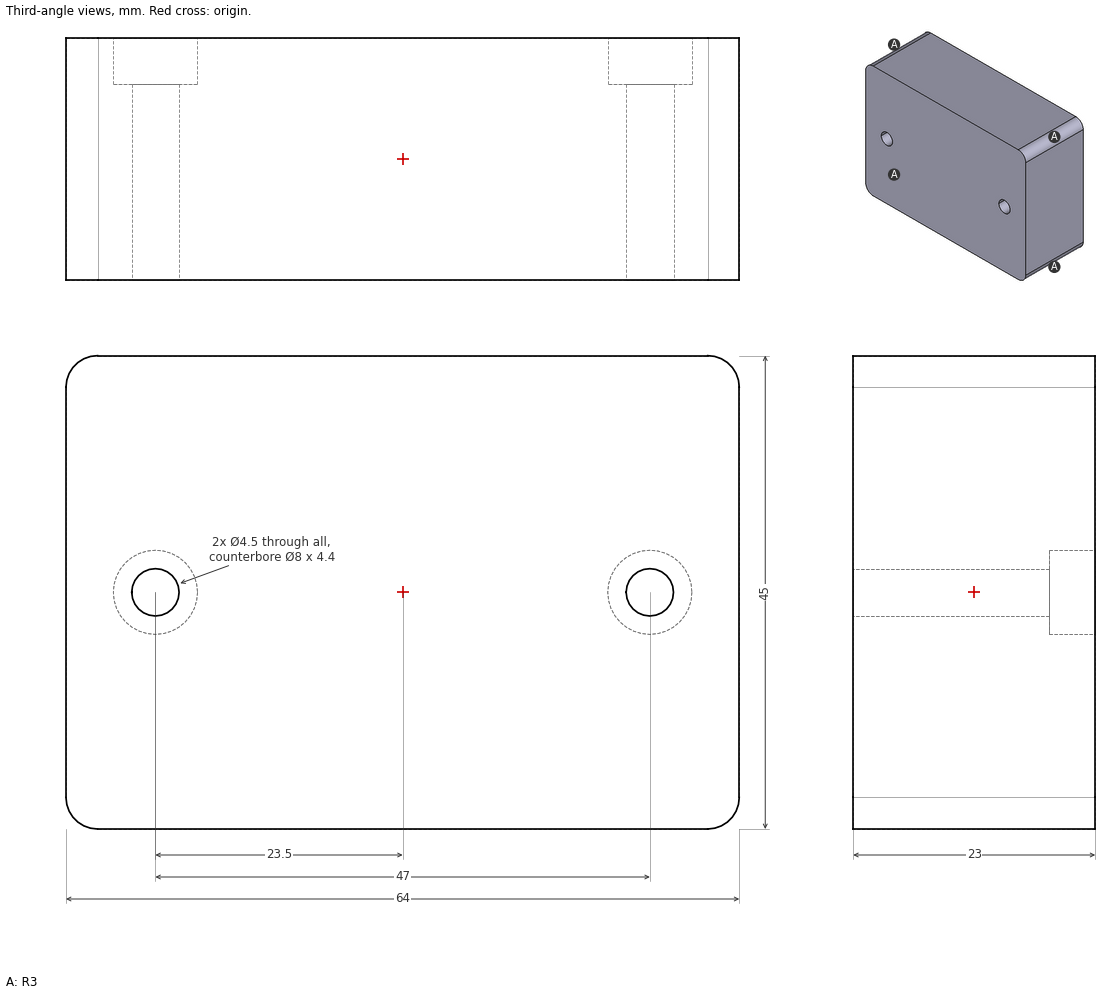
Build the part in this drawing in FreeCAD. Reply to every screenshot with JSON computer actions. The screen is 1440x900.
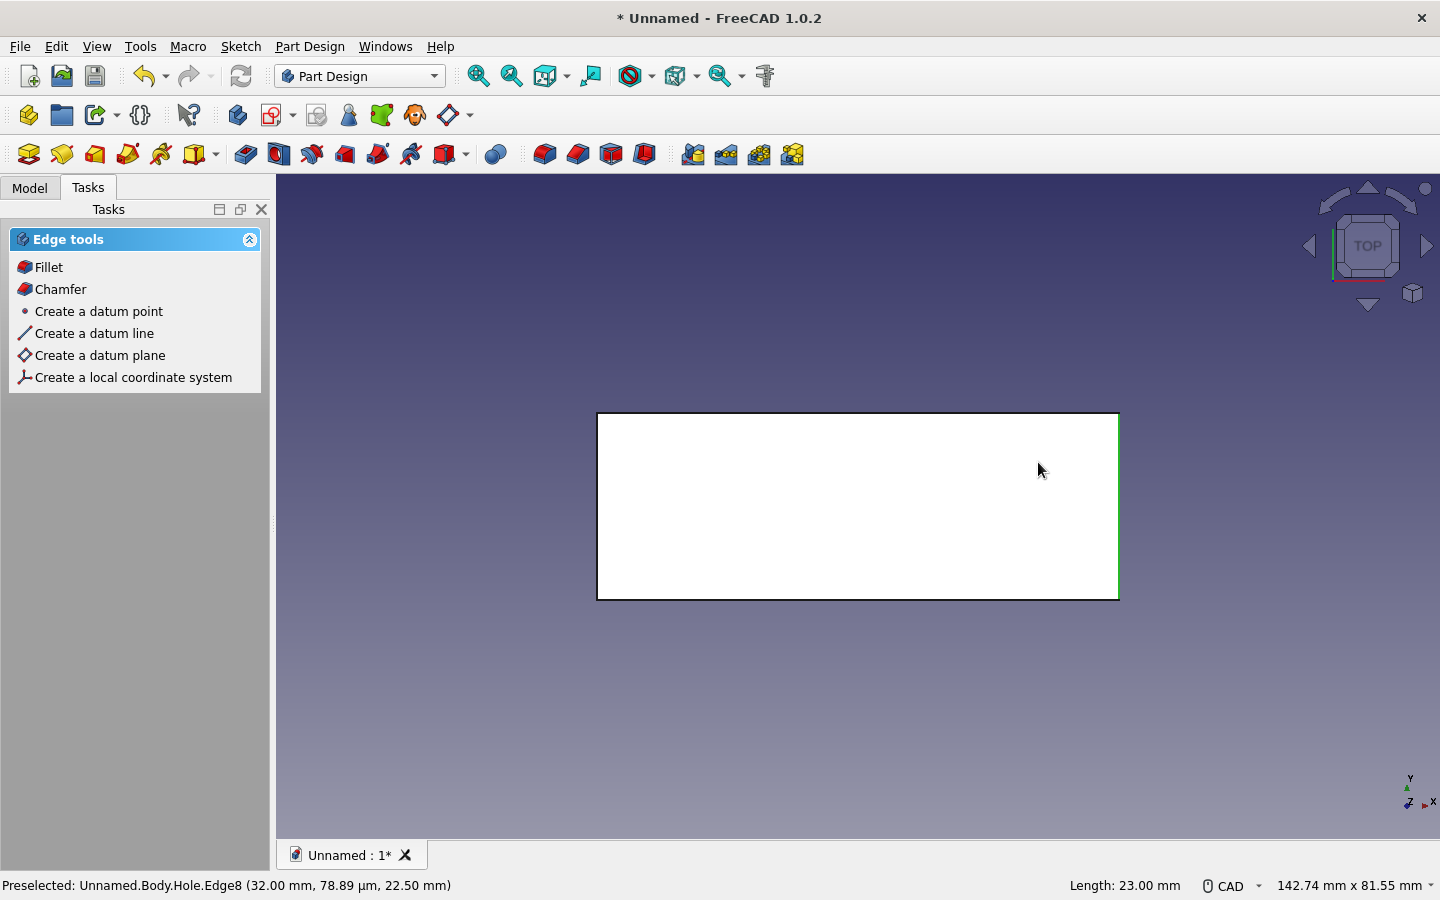
{"action": "left_click", "coordinate": [479, 76]}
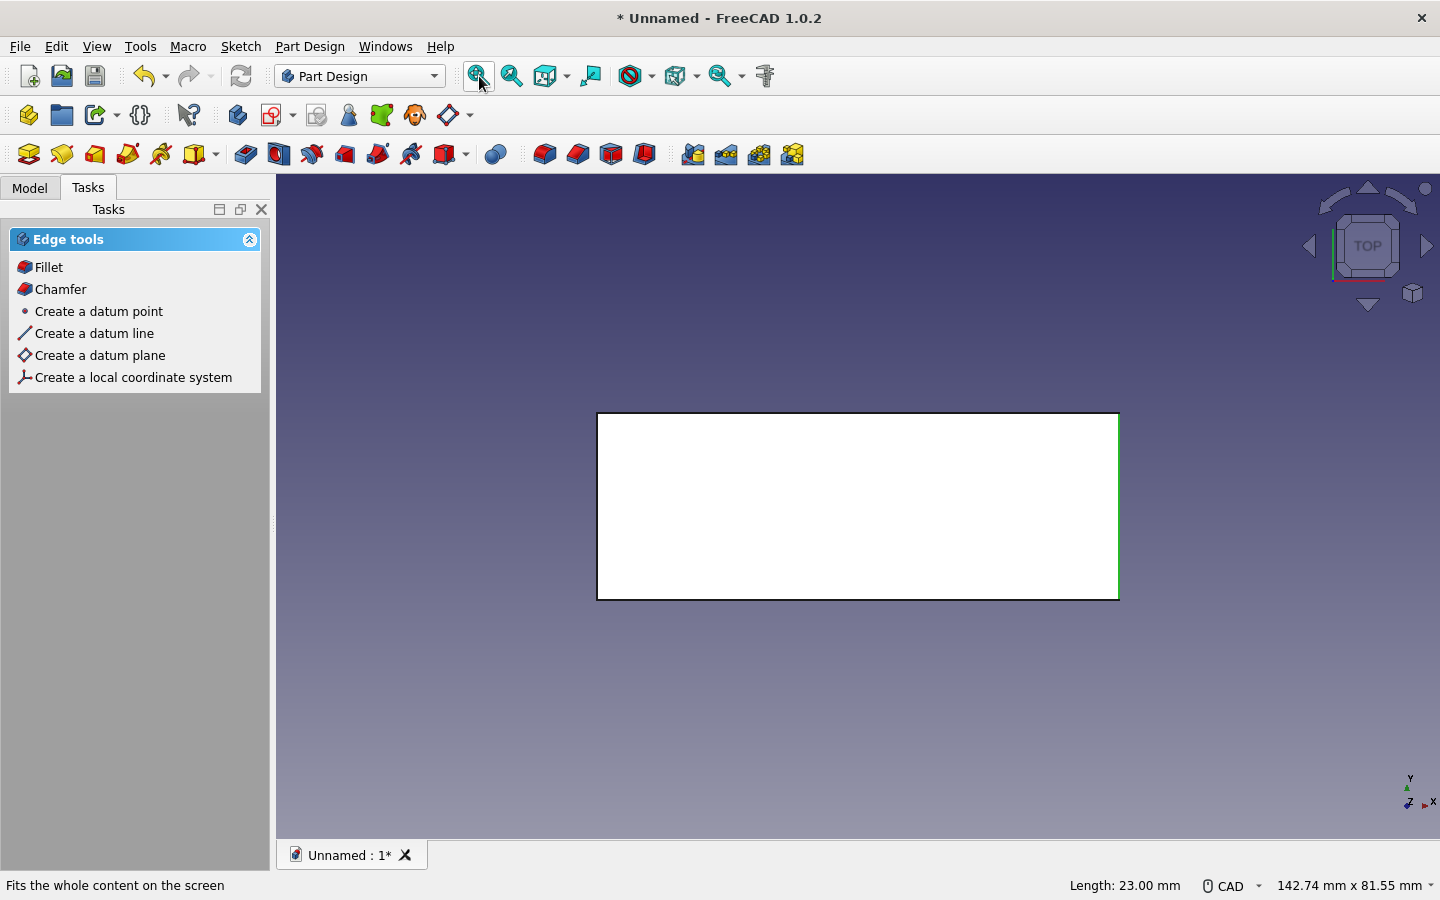
{"action": "left_click", "coordinate": [597, 505], "text": "ctrl"}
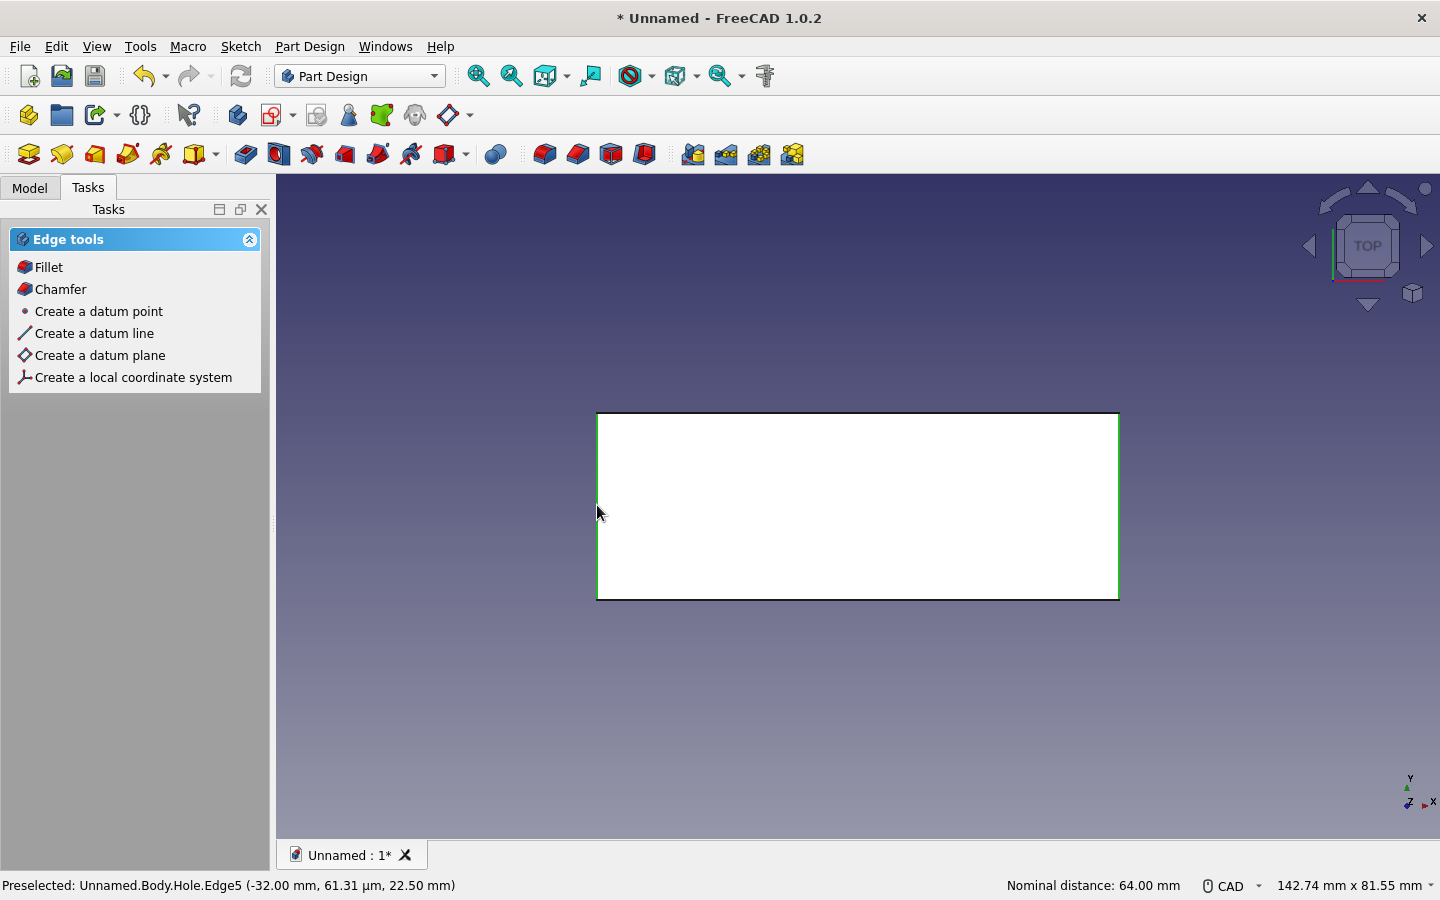
{"action": "key", "text": "1"}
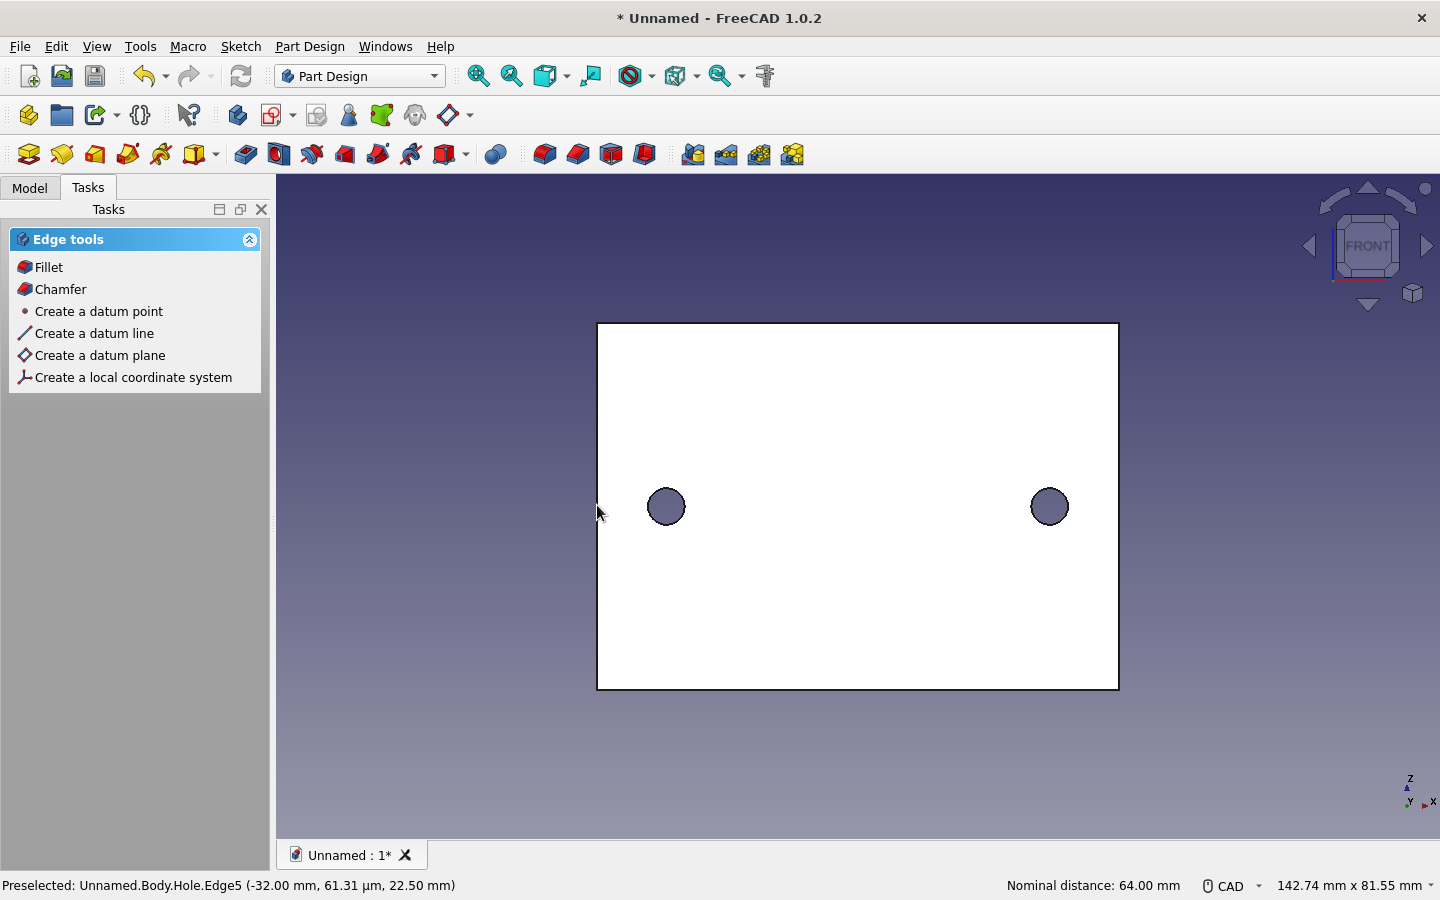
{"action": "key", "text": "3"}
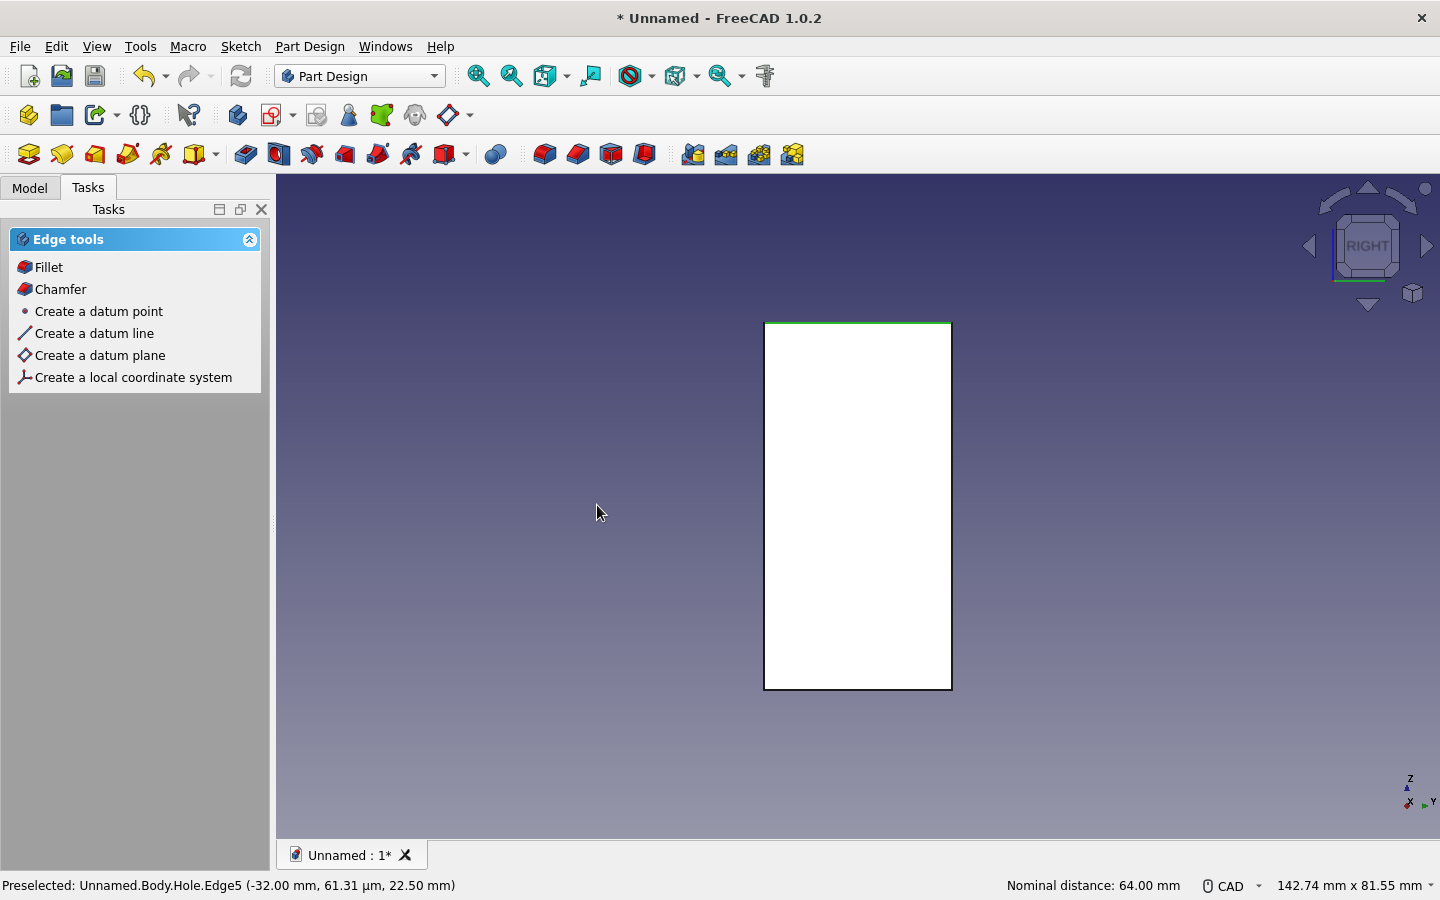
{"action": "left_click", "coordinate": [858, 689], "text": "ctrl"}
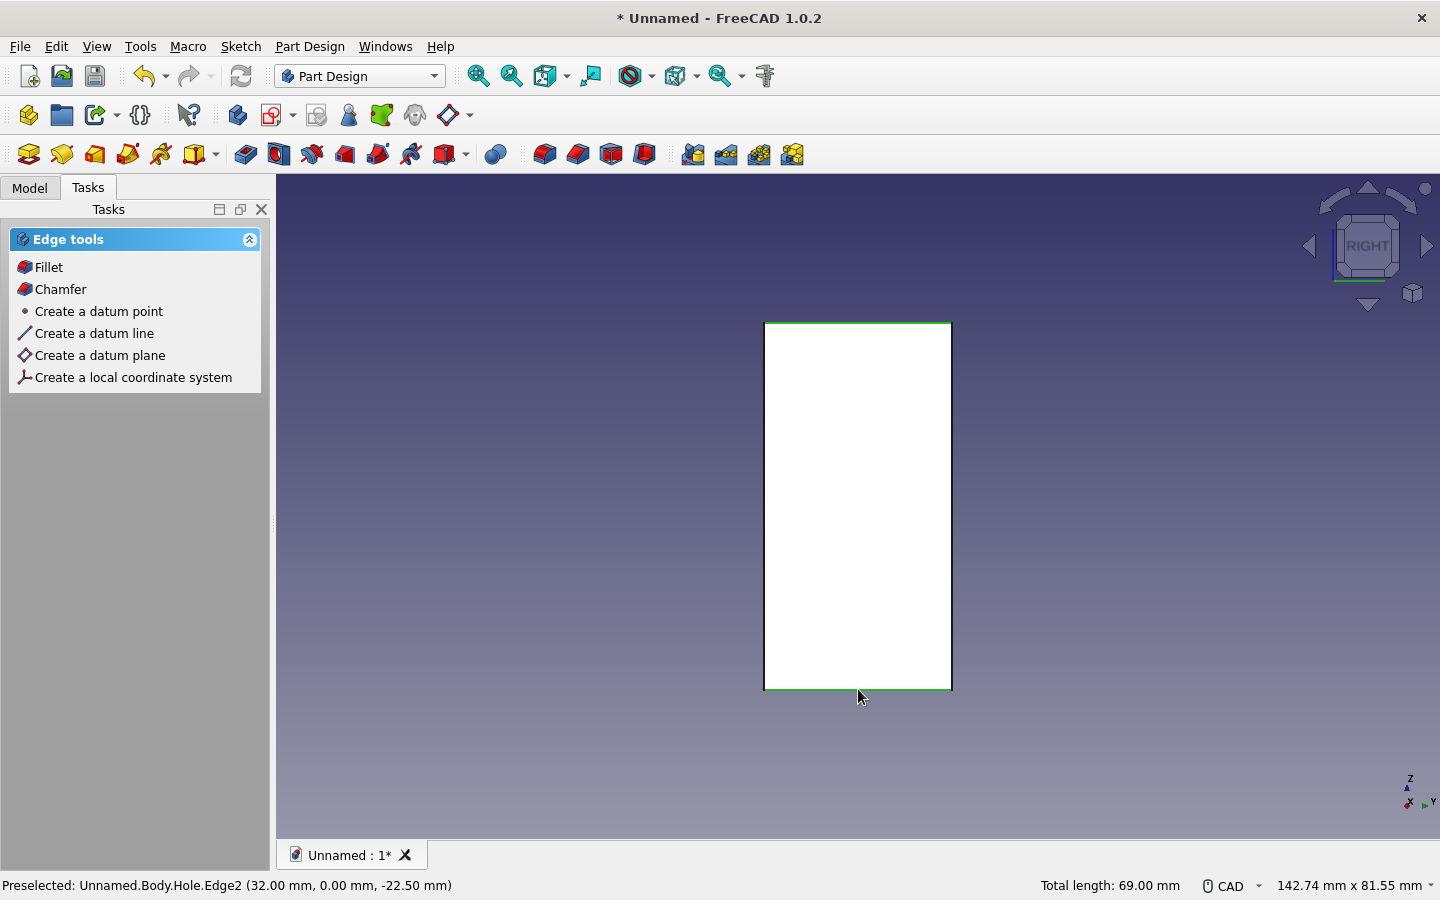
{"action": "key", "text": "5"}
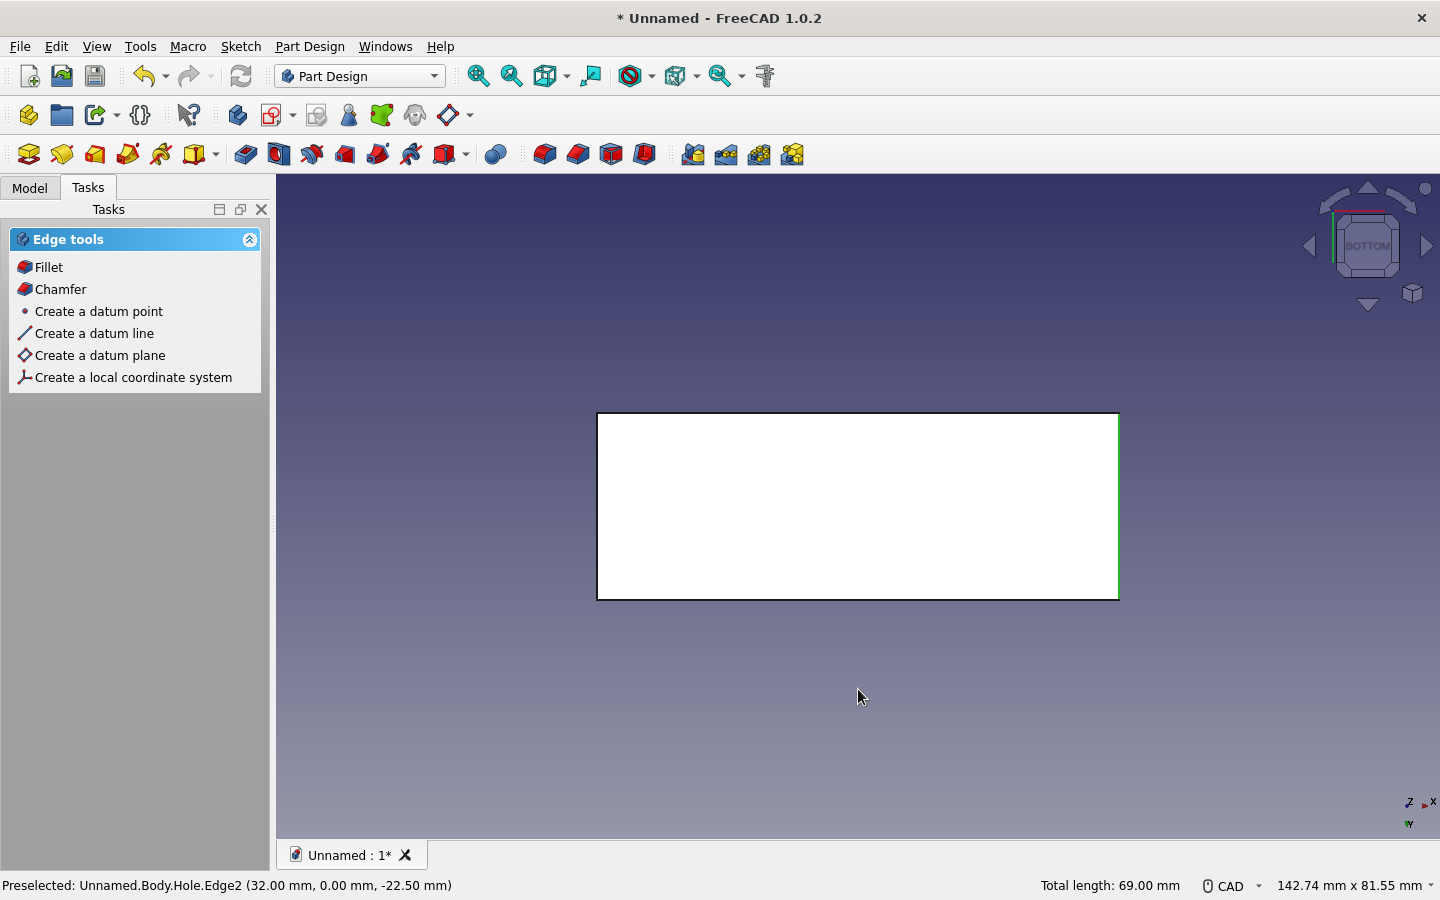
{"action": "left_click", "coordinate": [479, 76]}